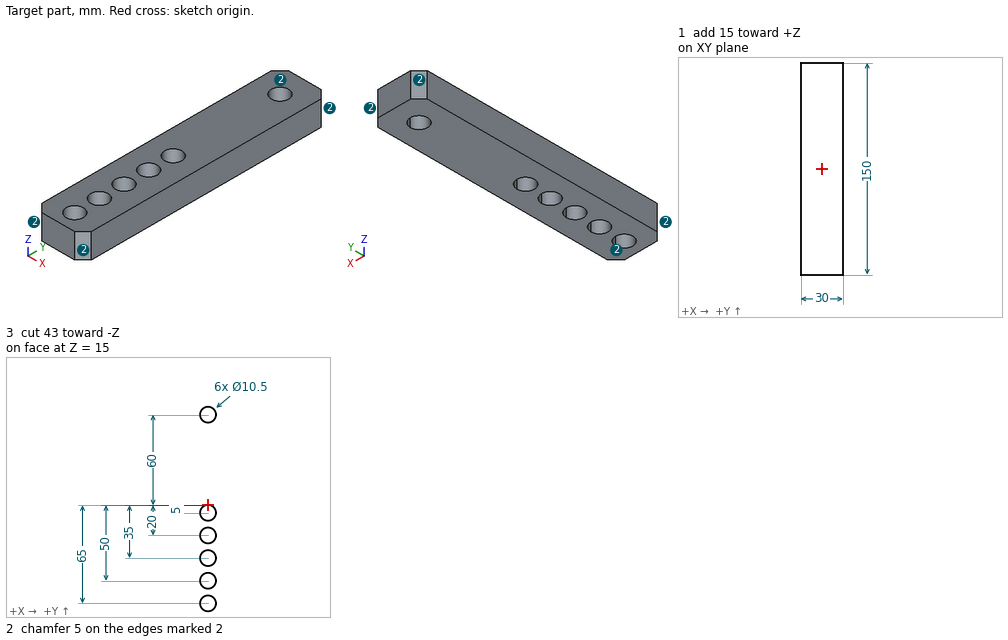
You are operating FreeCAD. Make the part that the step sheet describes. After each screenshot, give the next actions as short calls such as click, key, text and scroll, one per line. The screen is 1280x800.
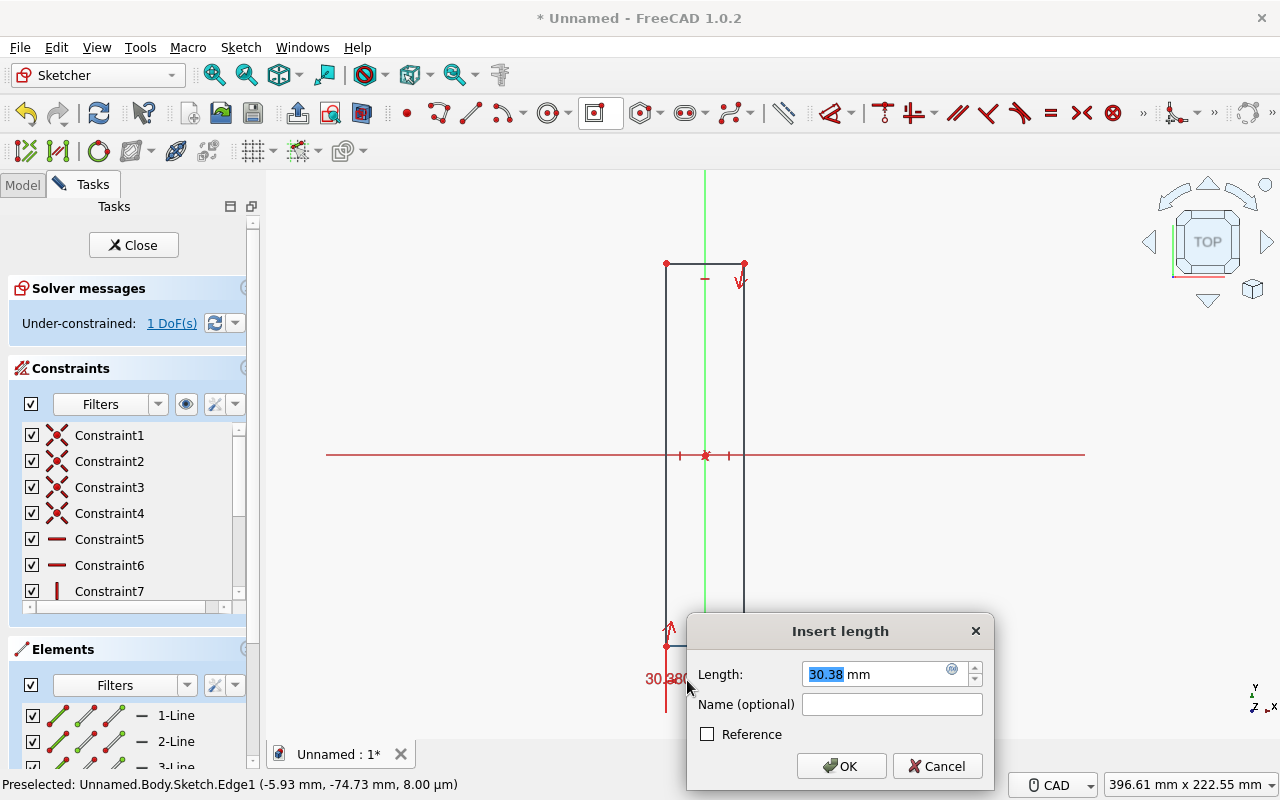
text(30)
key(Return)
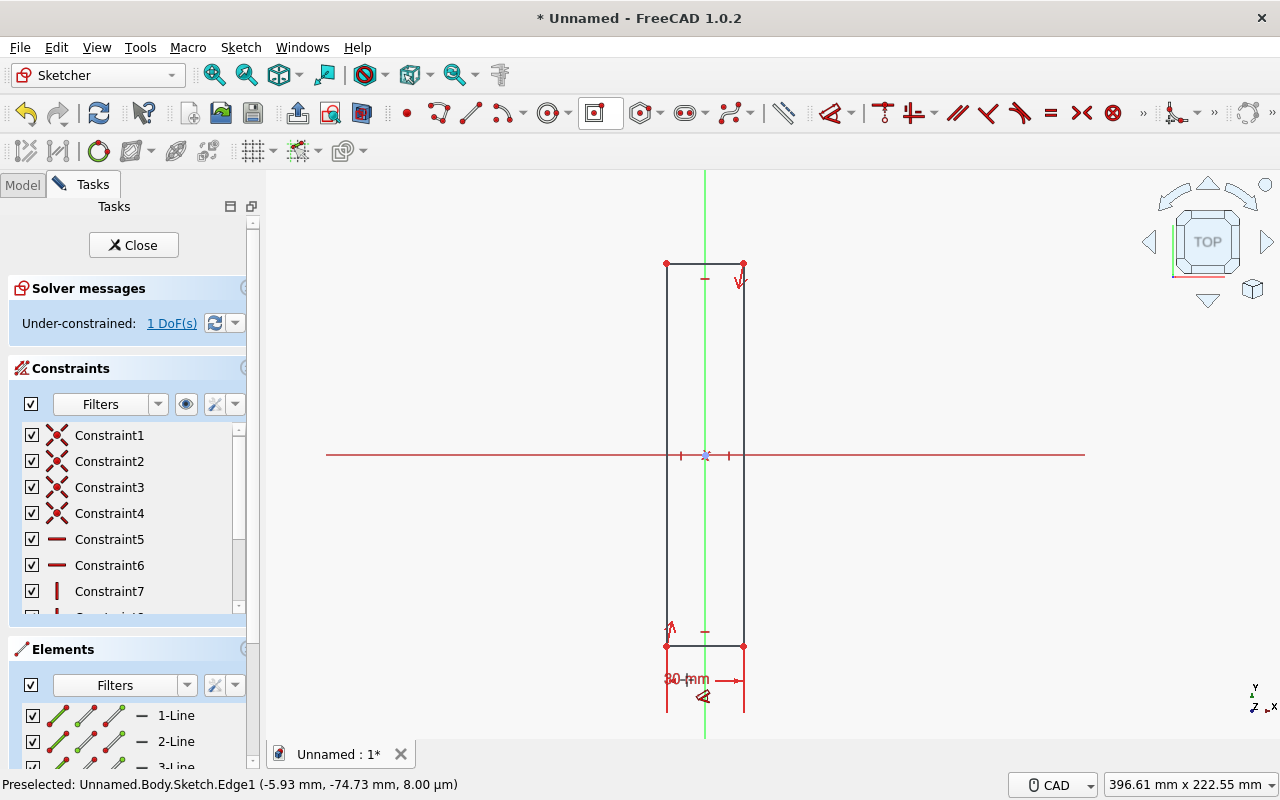
click(744, 531)
click(778, 367)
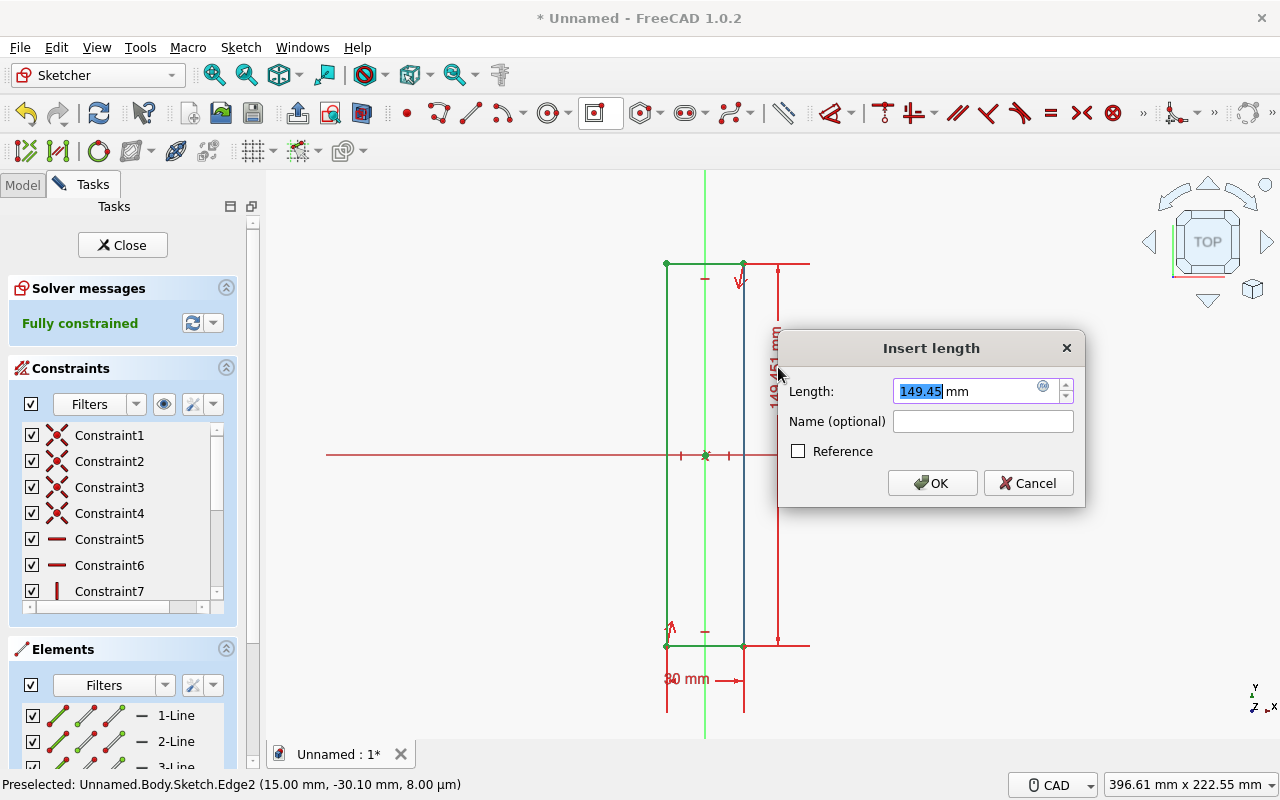
text(150)
key(Return)
key(Escape)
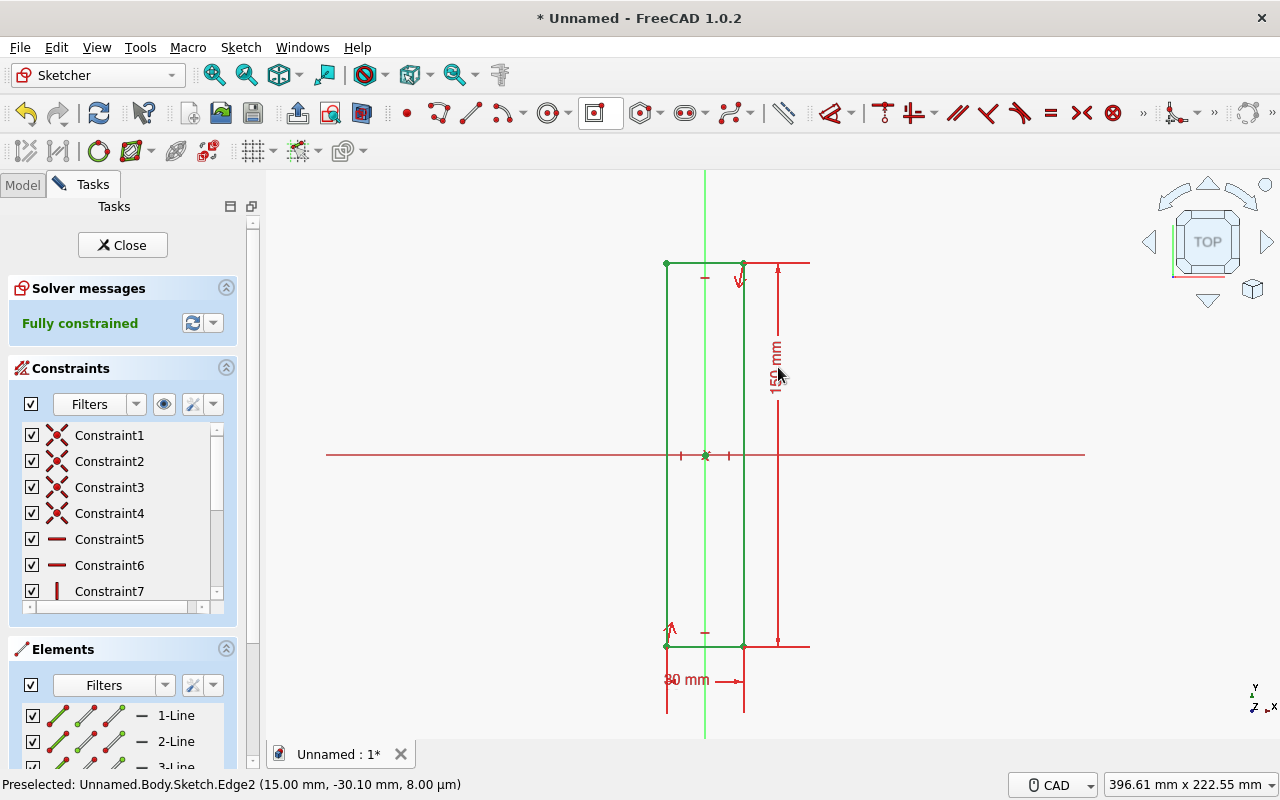
click(123, 245)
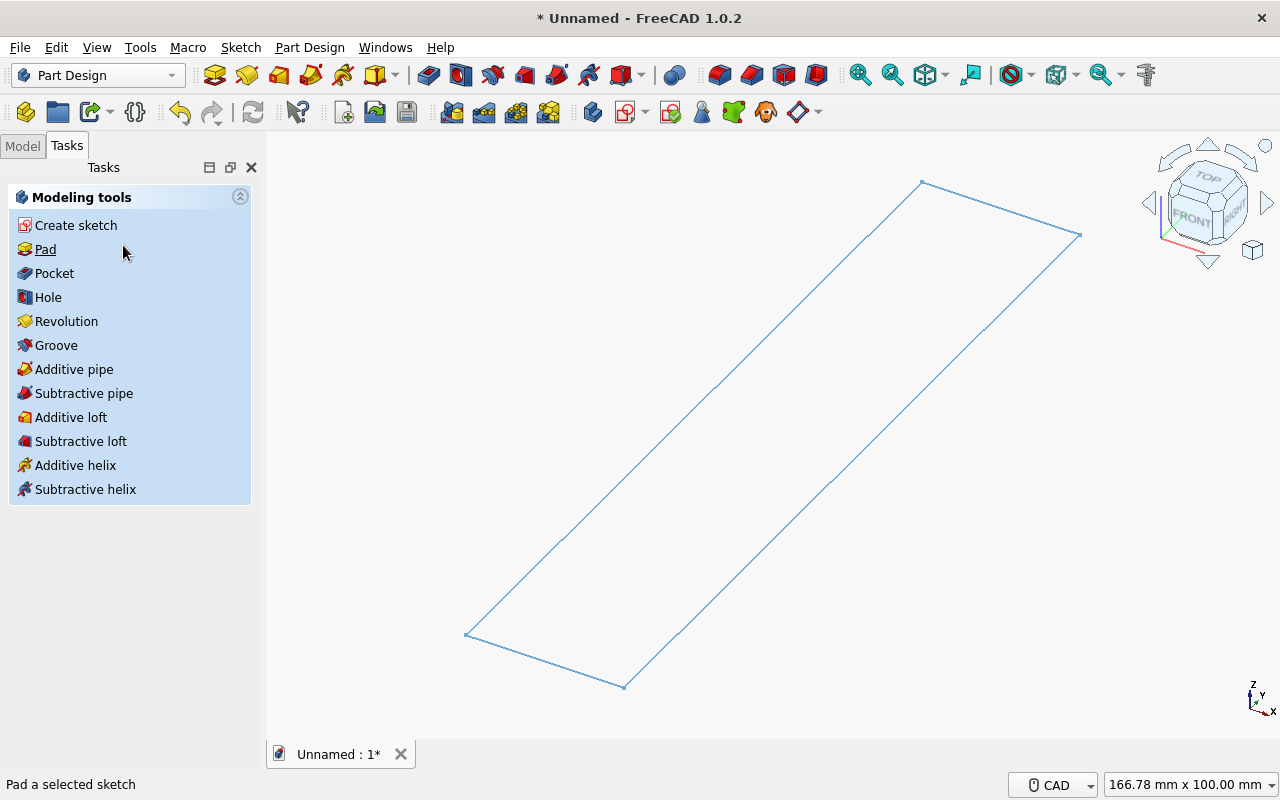
click(216, 76)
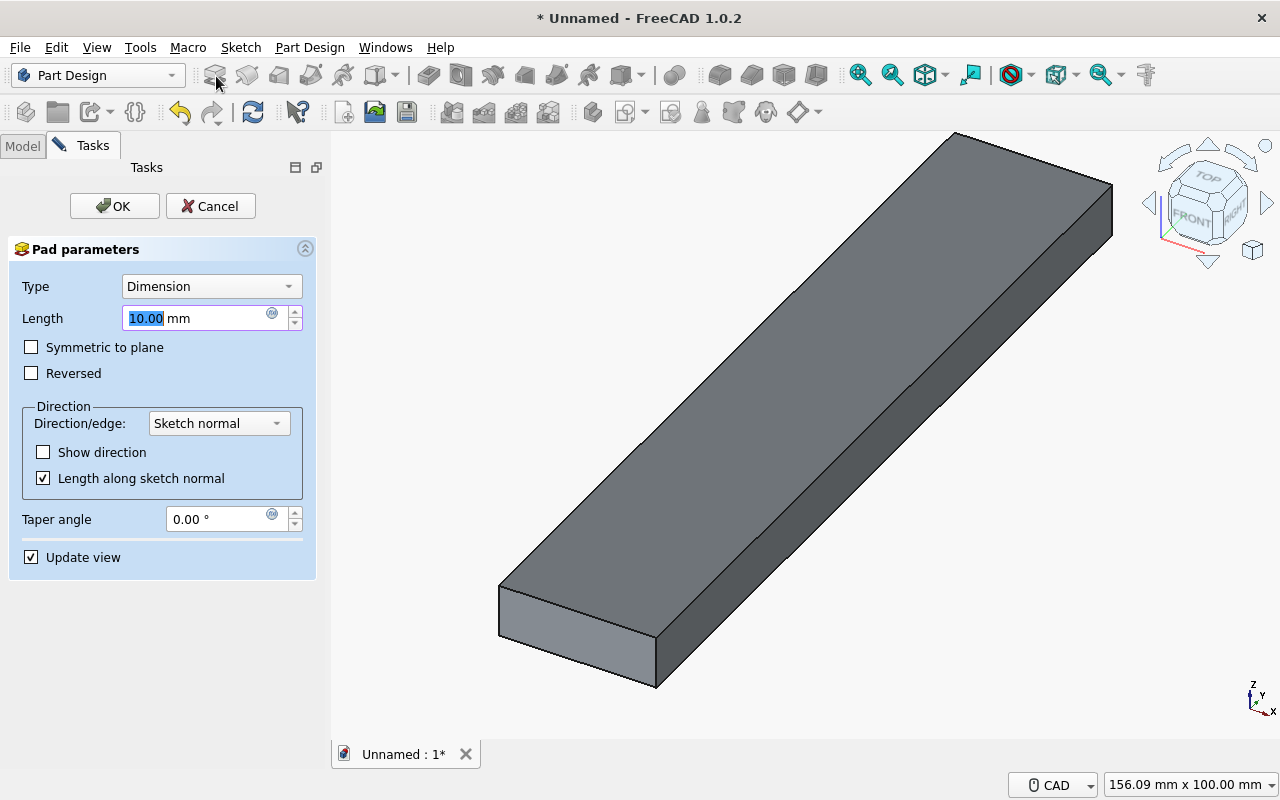
text(15)
key(Tab)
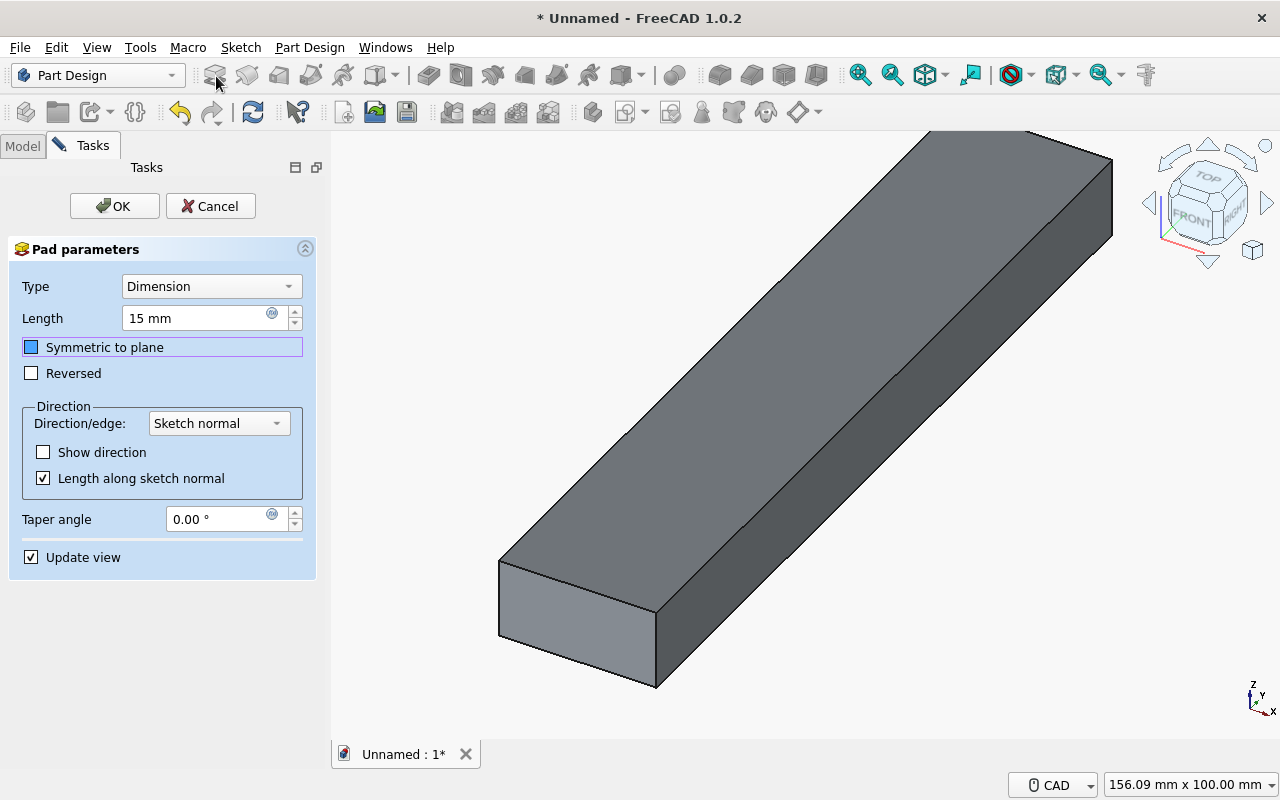
click(115, 206)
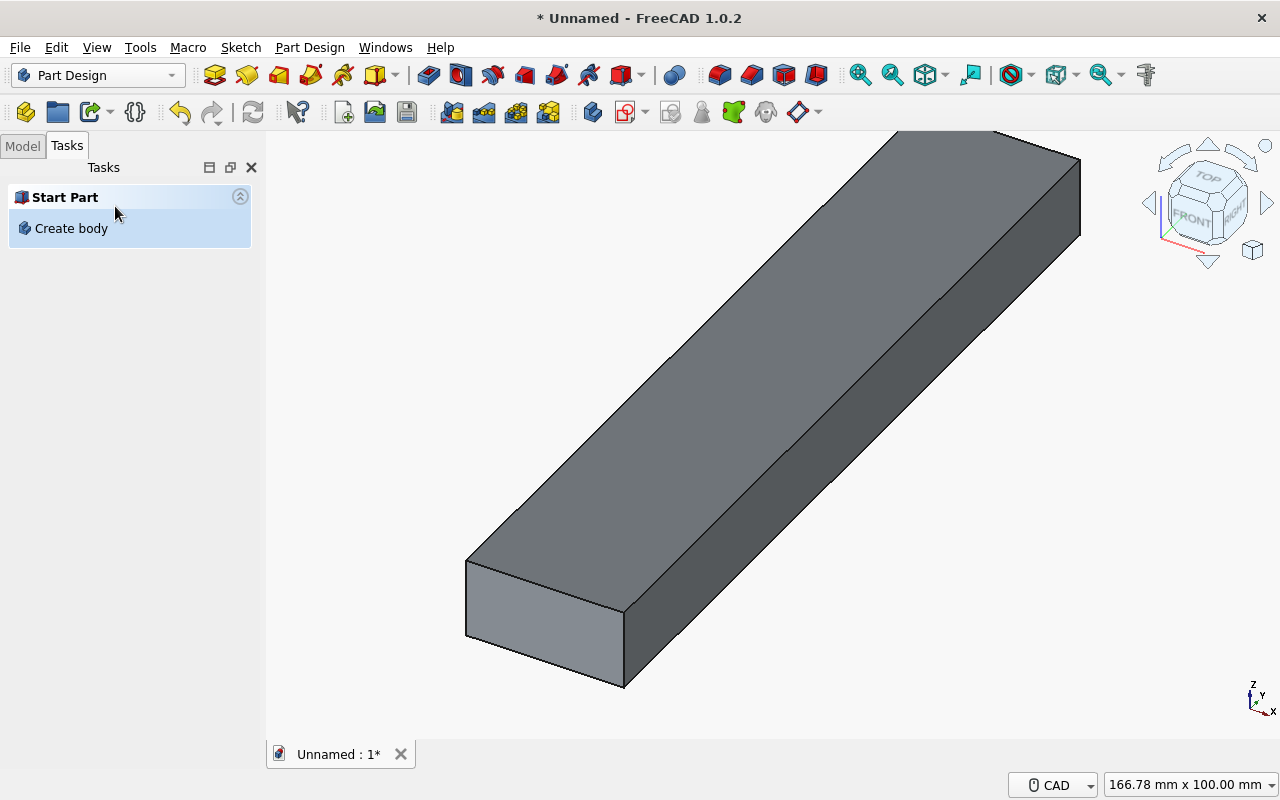
click(862, 76)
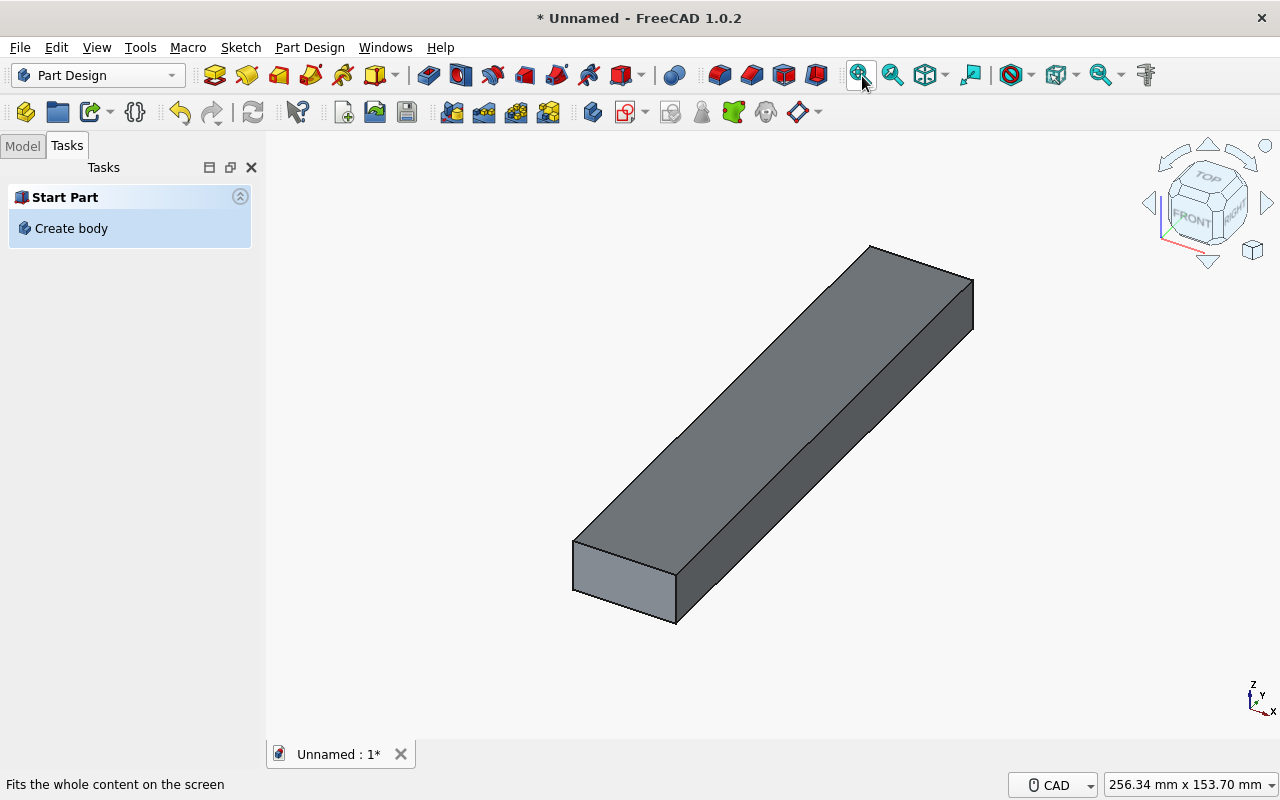
click(676, 598)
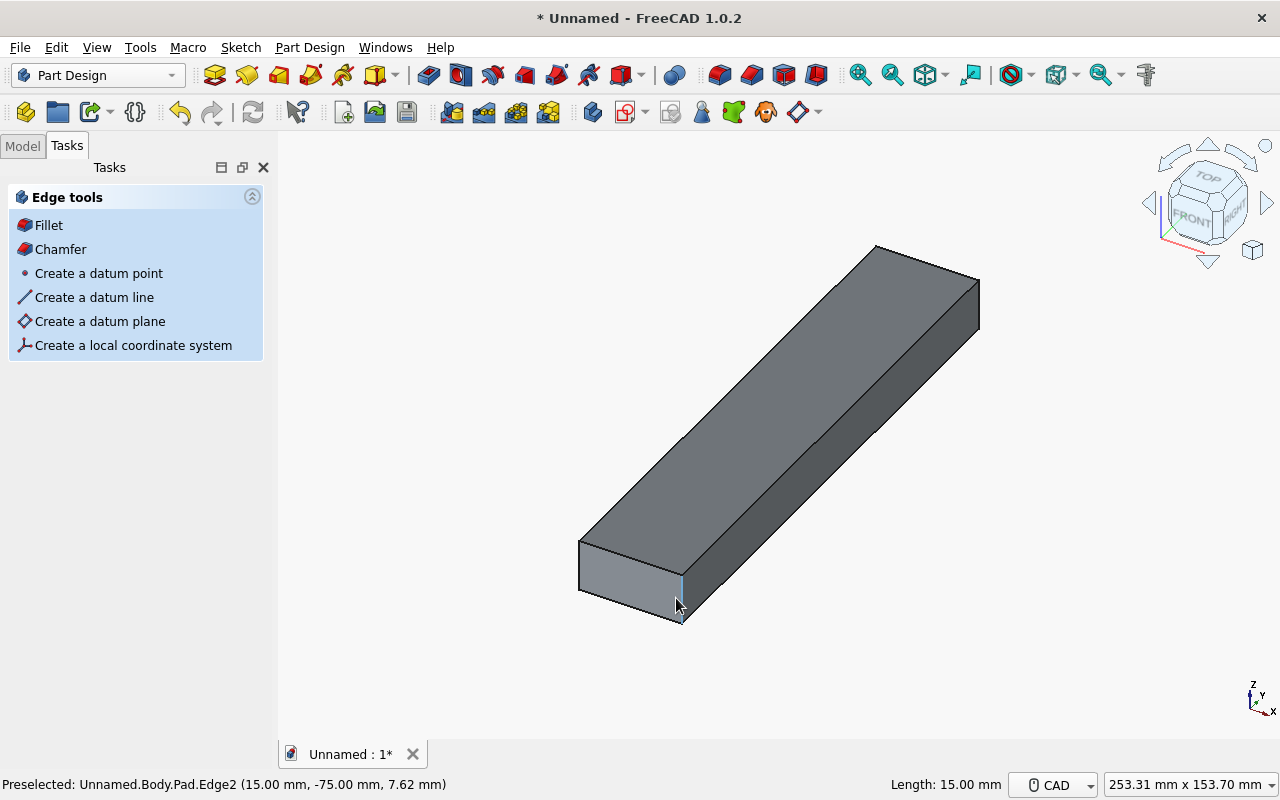
key(0)